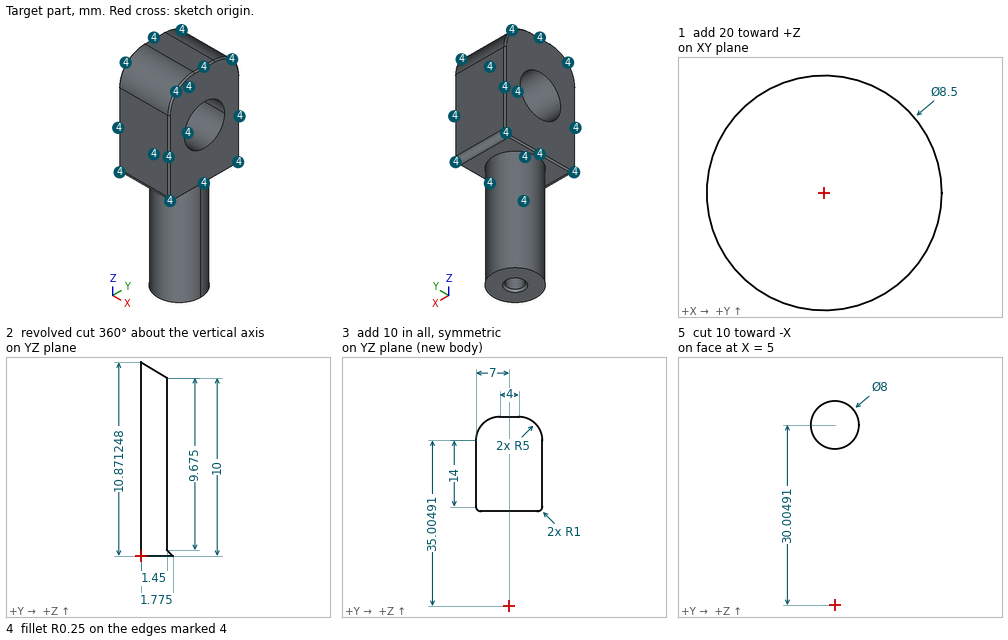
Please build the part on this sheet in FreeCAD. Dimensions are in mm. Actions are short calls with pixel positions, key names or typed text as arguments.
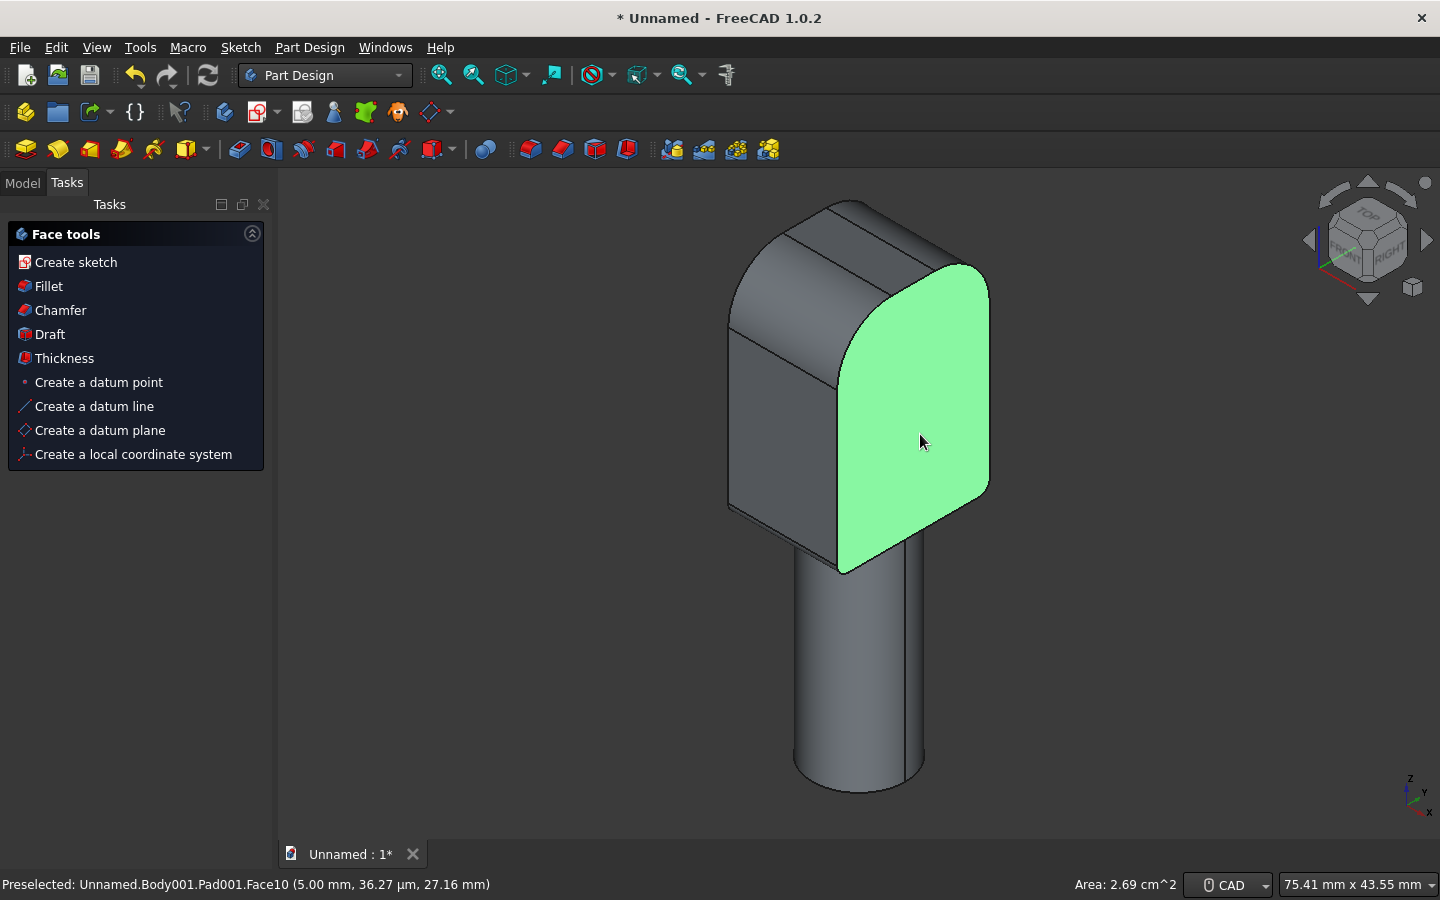
key(2)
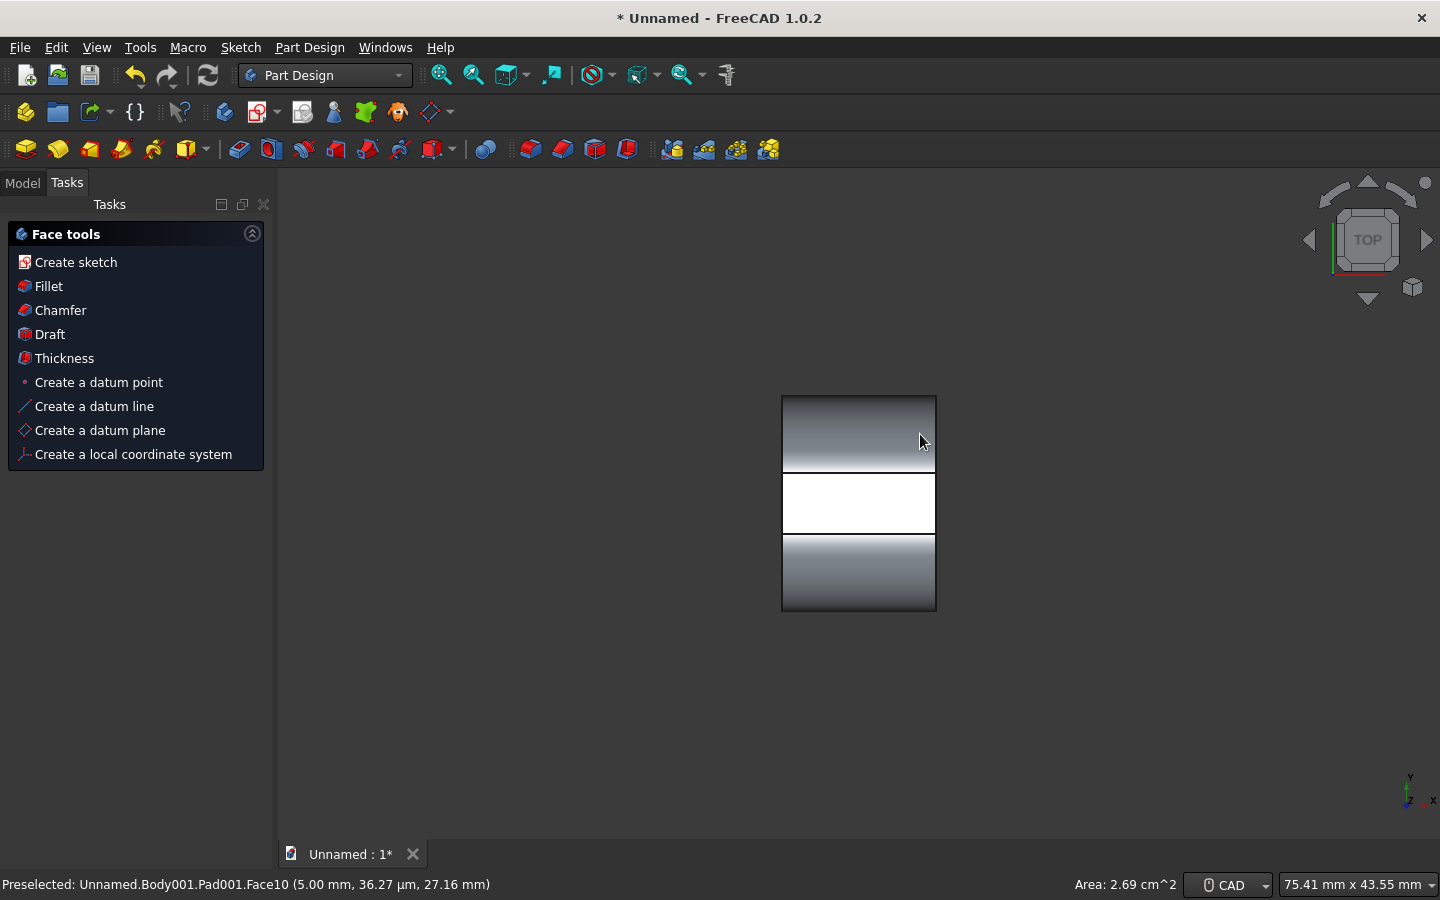
click(442, 76)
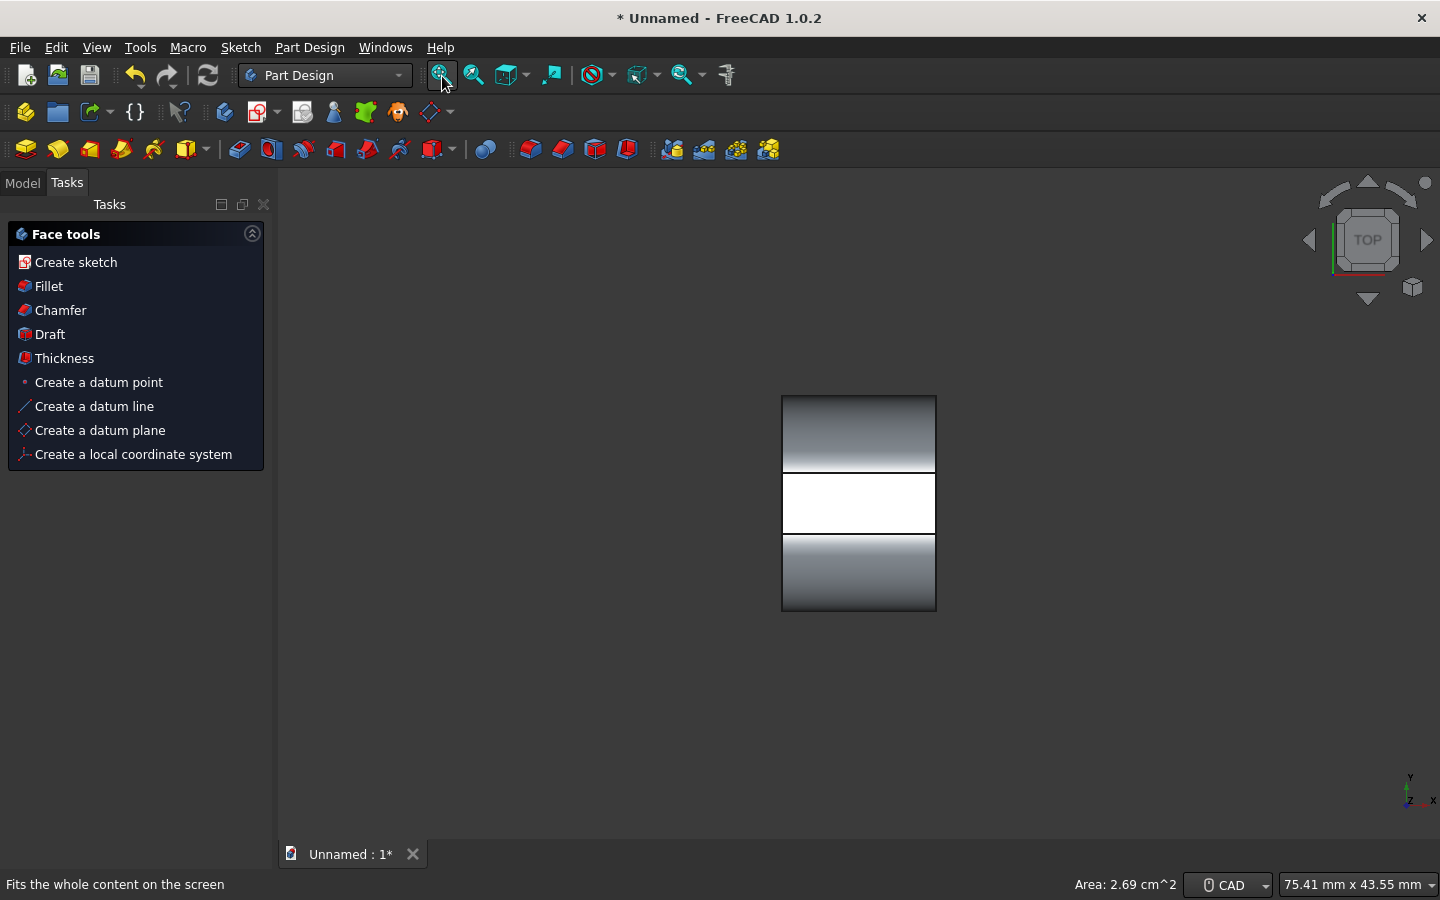
key(1)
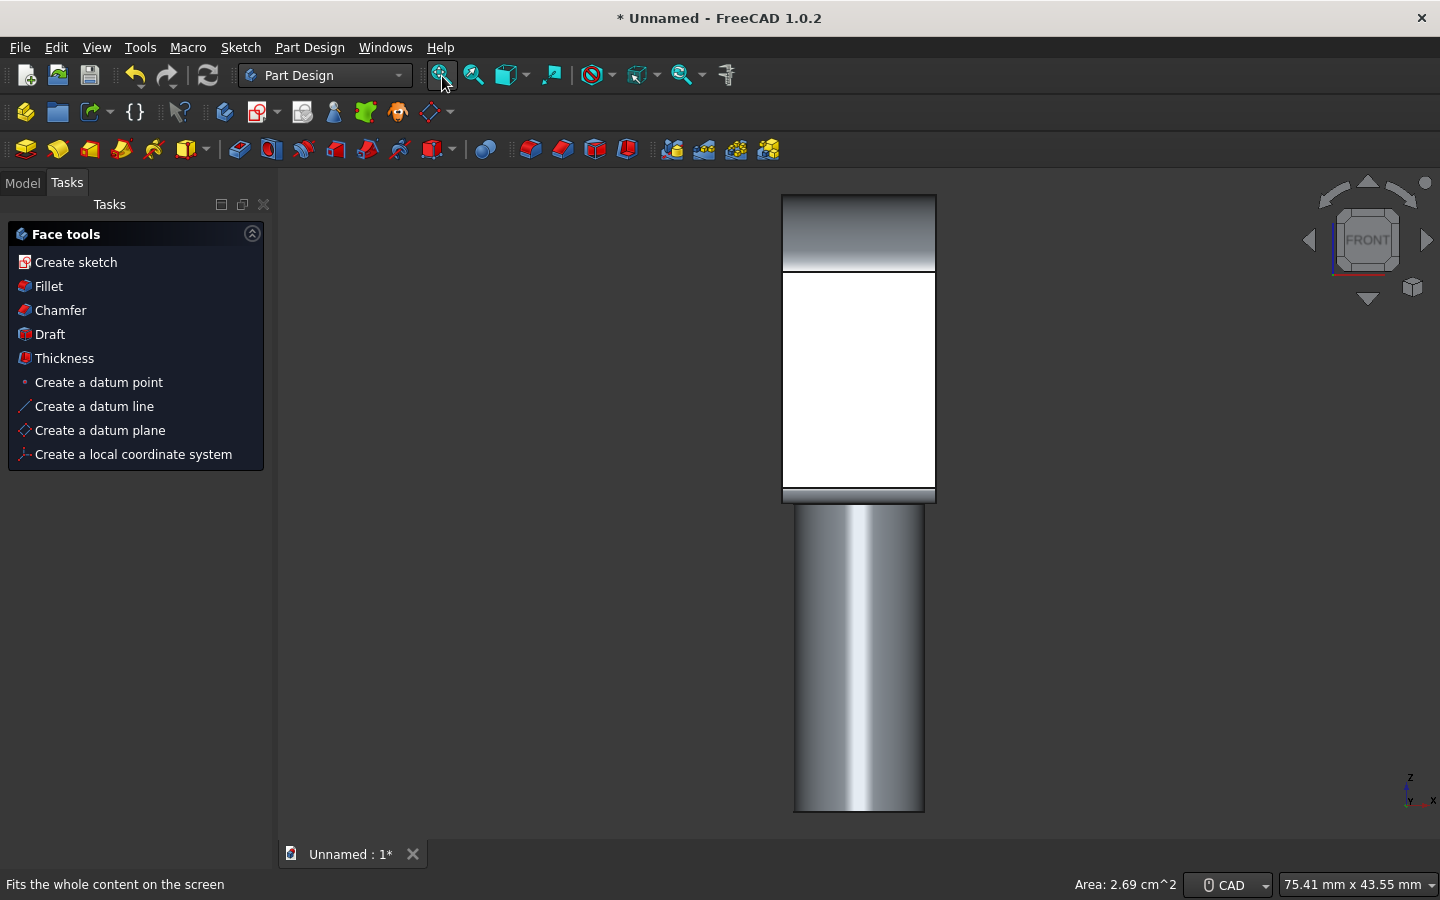
key(3)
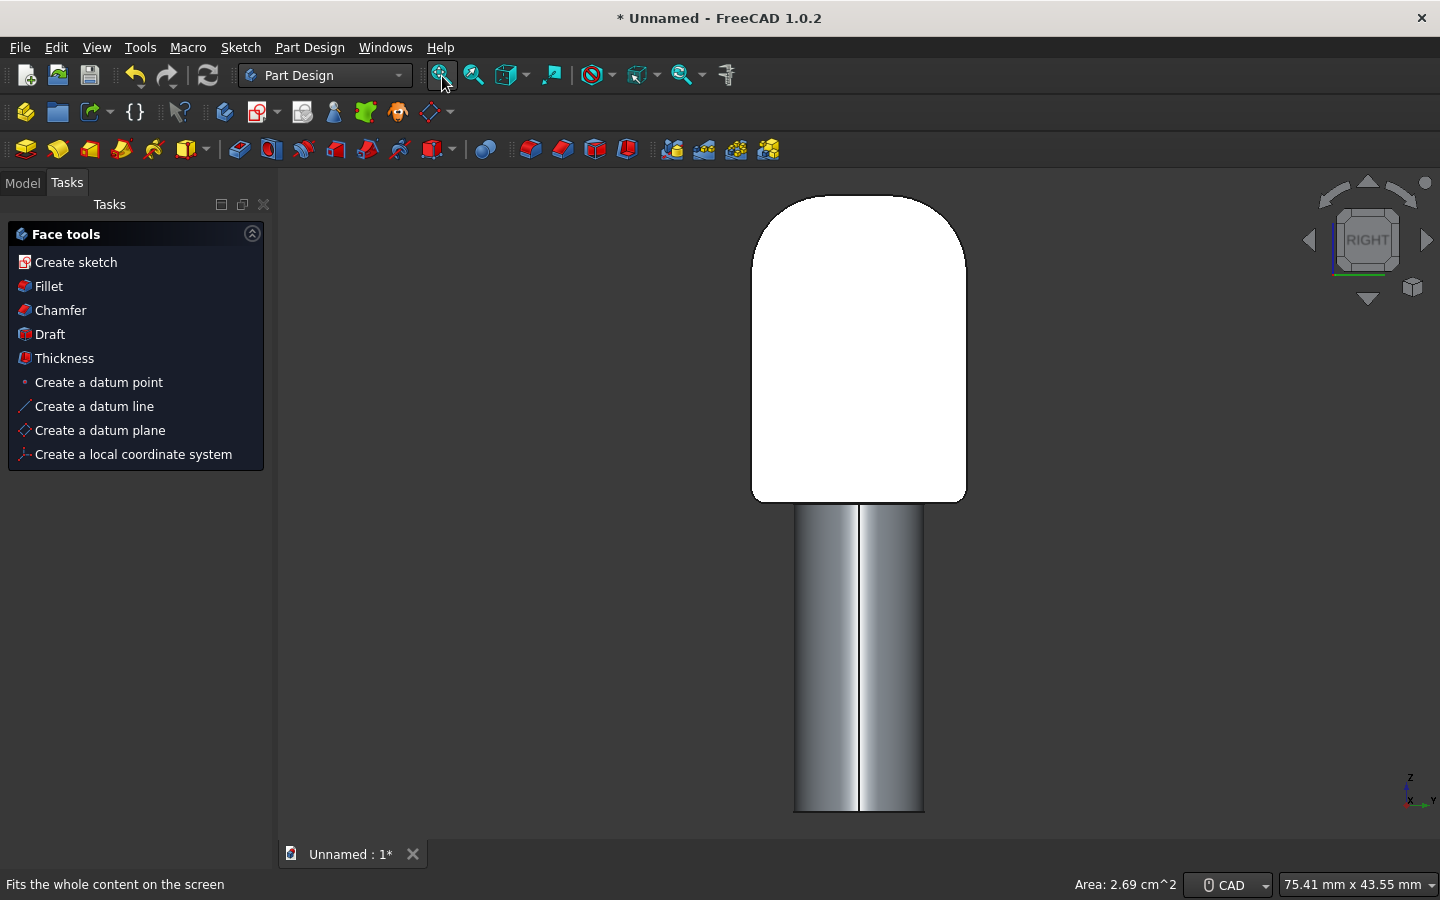
key(5)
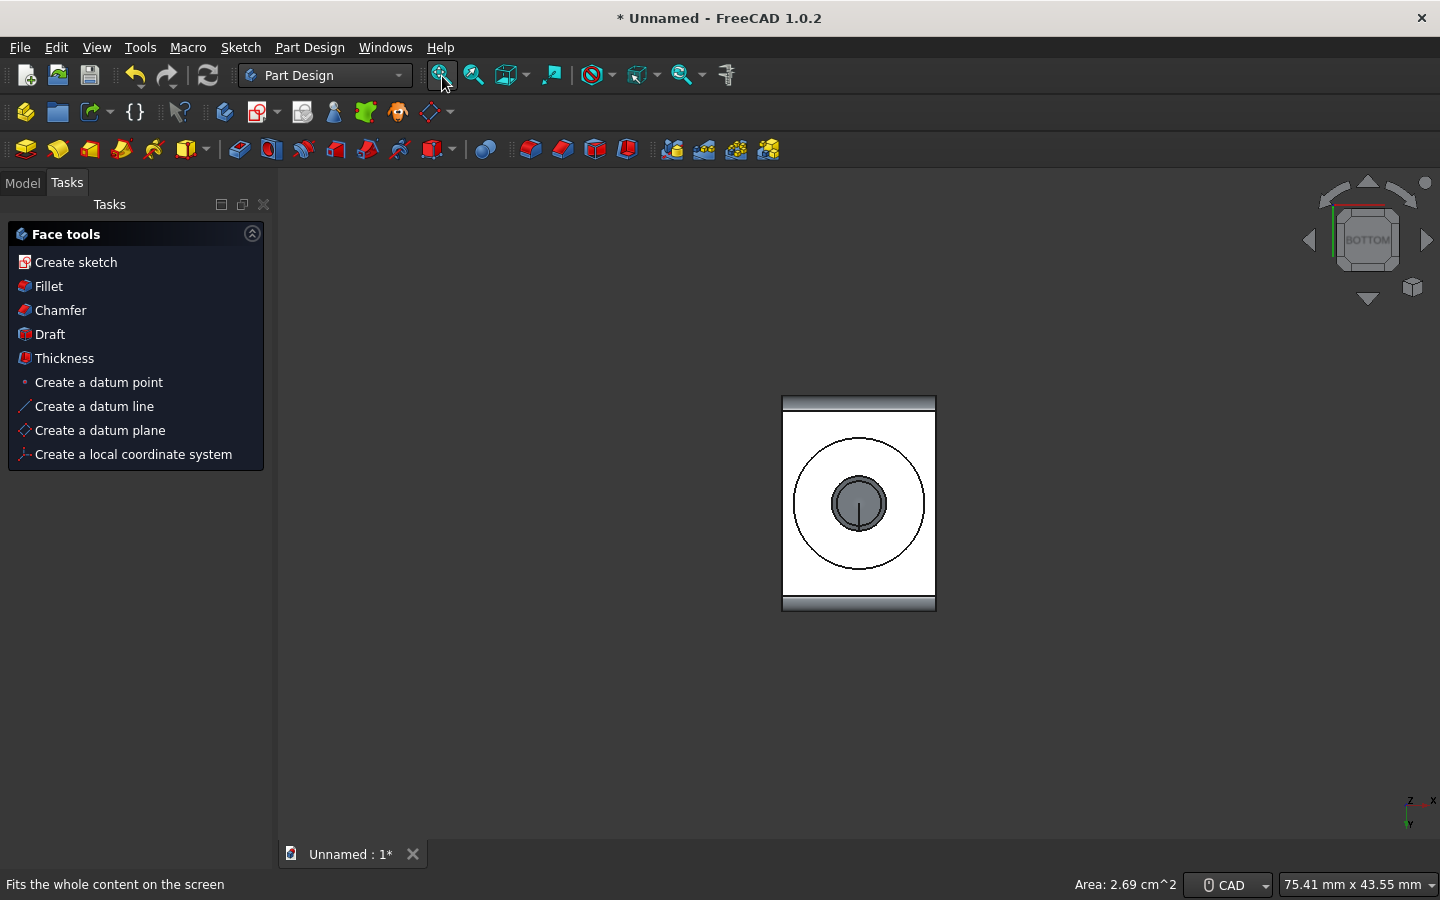
click(442, 76)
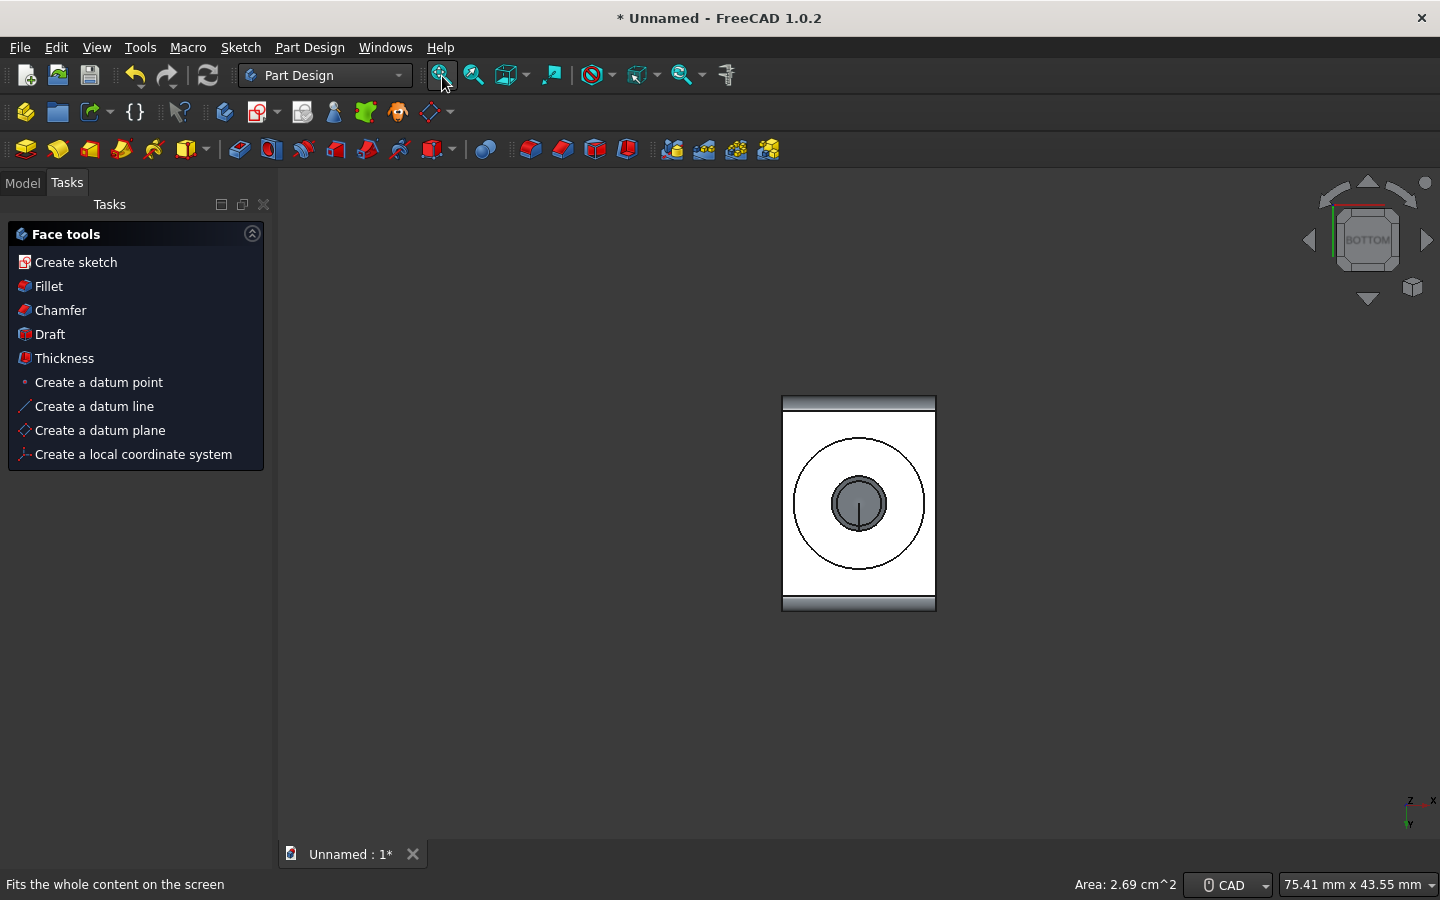
key(4)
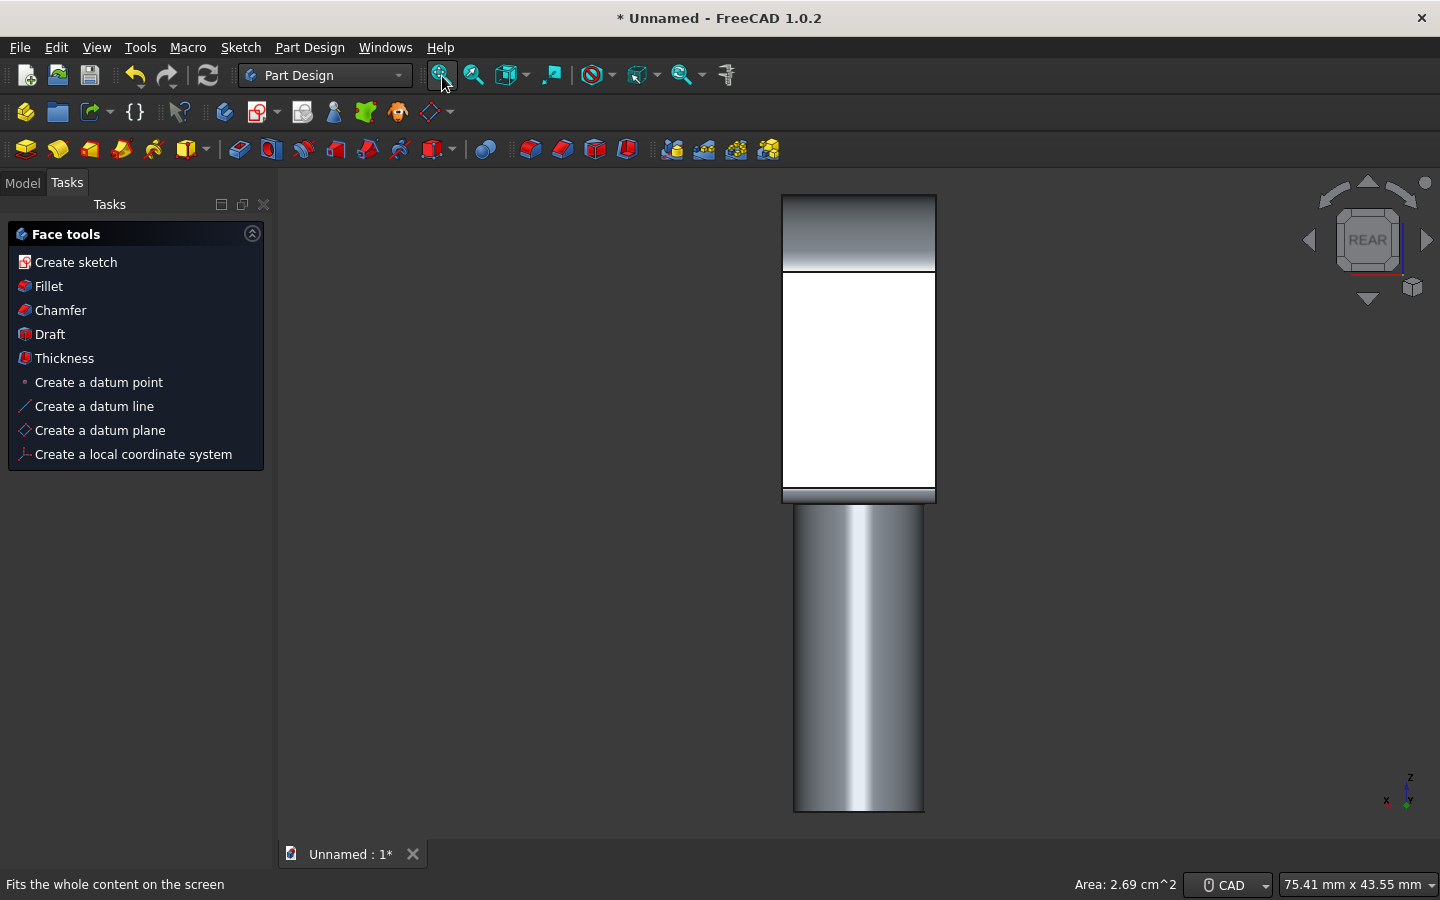
key(6)